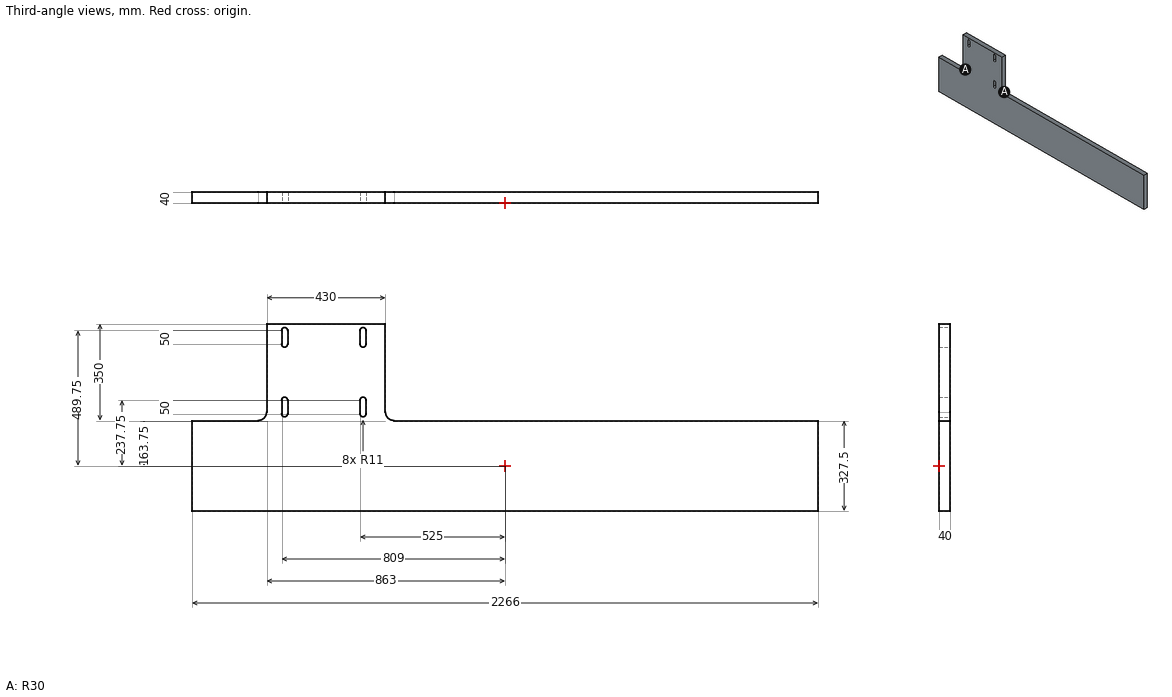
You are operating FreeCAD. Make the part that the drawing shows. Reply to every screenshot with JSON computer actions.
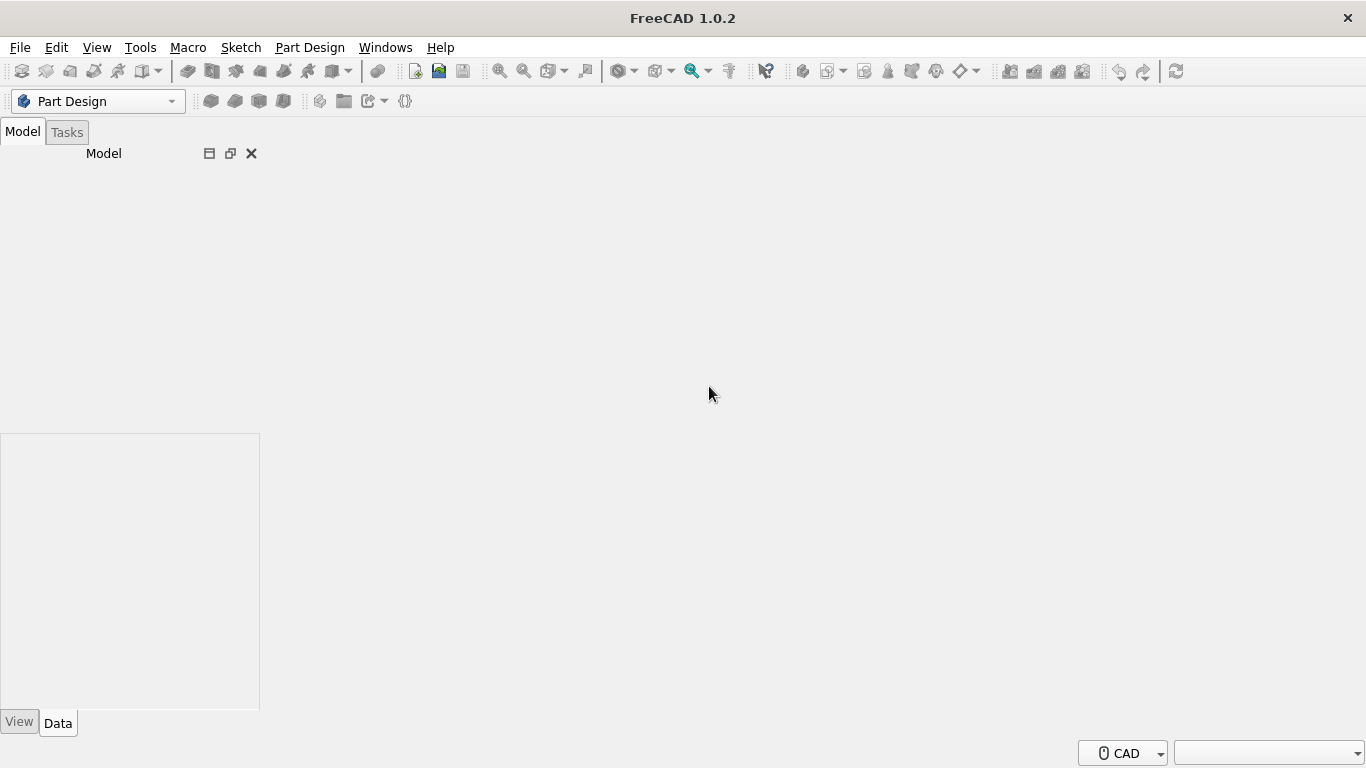
{"action": "left_click", "coordinate": [416, 72]}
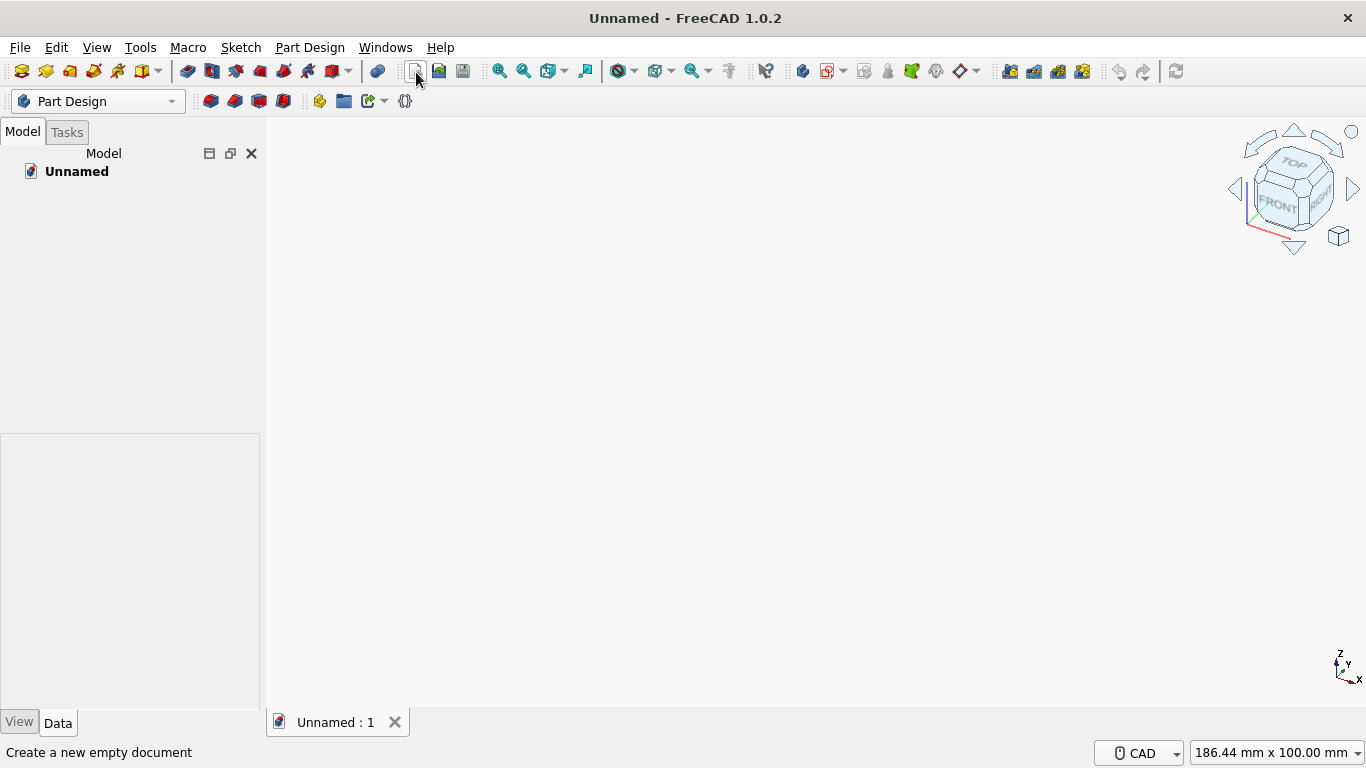
{"action": "left_click", "coordinate": [828, 72]}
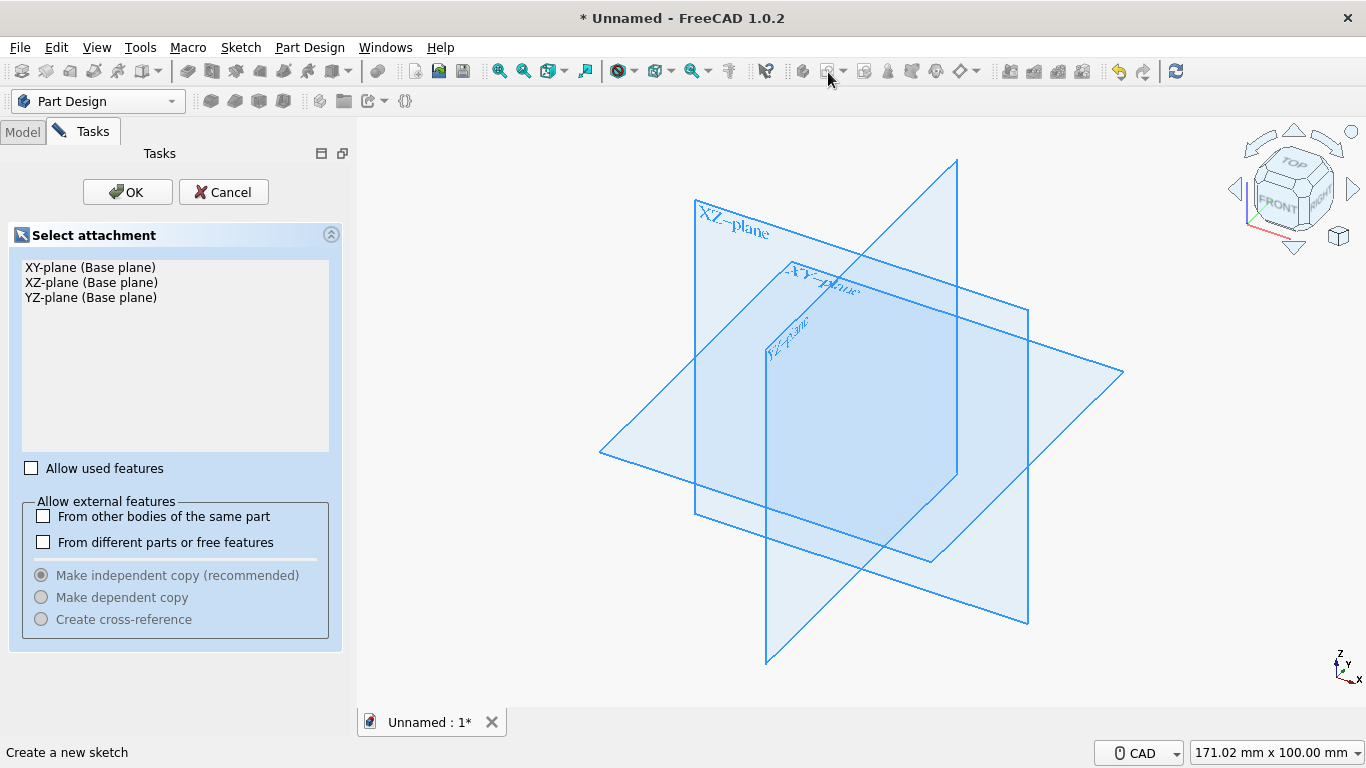
{"action": "left_click", "coordinate": [82, 282]}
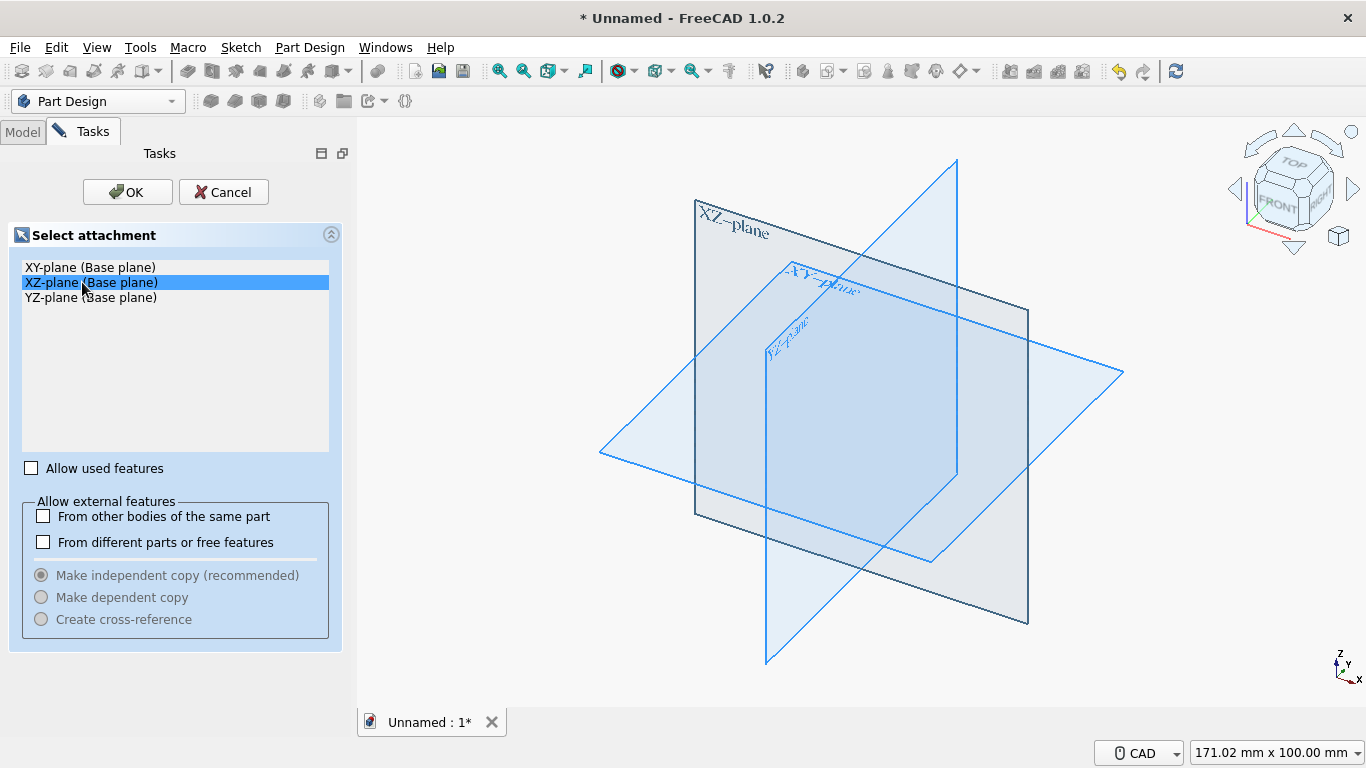
{"action": "left_click", "coordinate": [128, 192]}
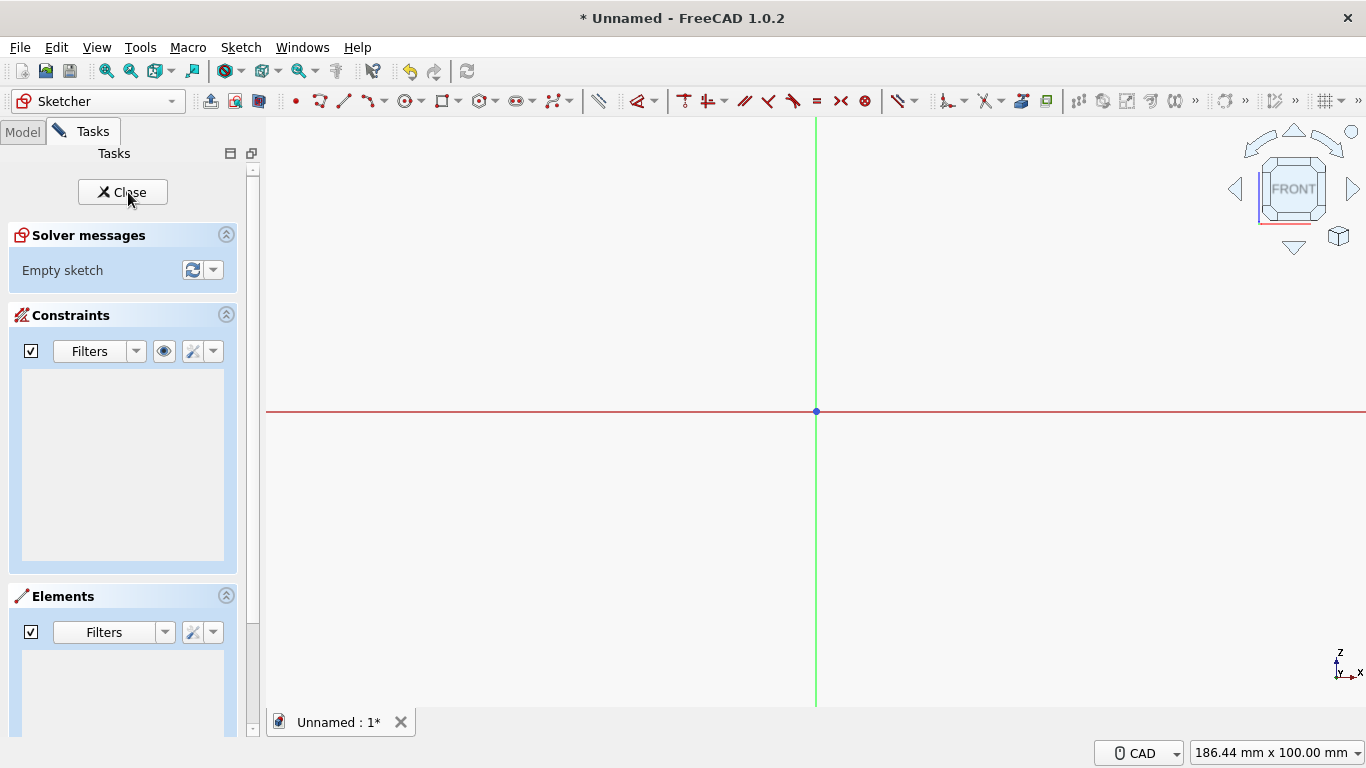
{"action": "scroll", "coordinate": [744, 412], "scroll_direction": "down", "scroll_amount": 15}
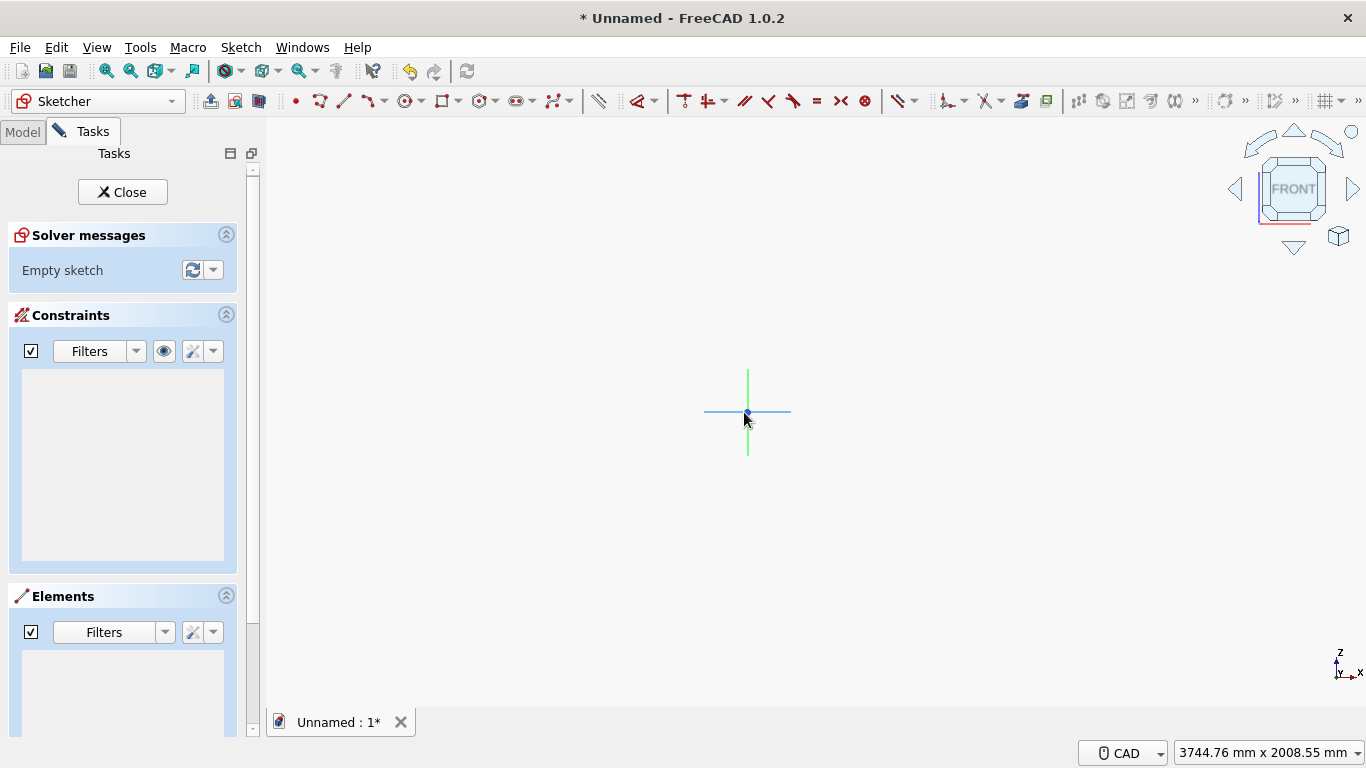
{"action": "left_click", "coordinate": [460, 102]}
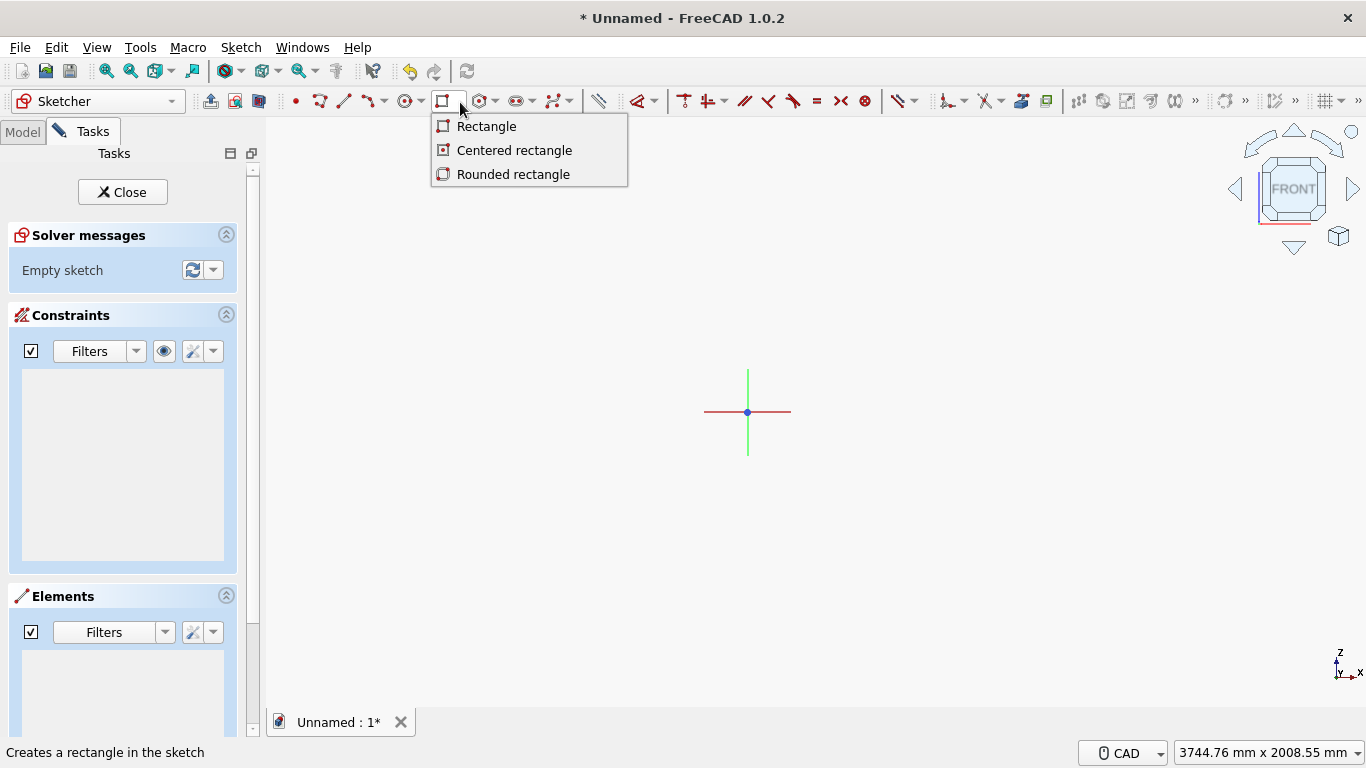
{"action": "left_click", "coordinate": [530, 150]}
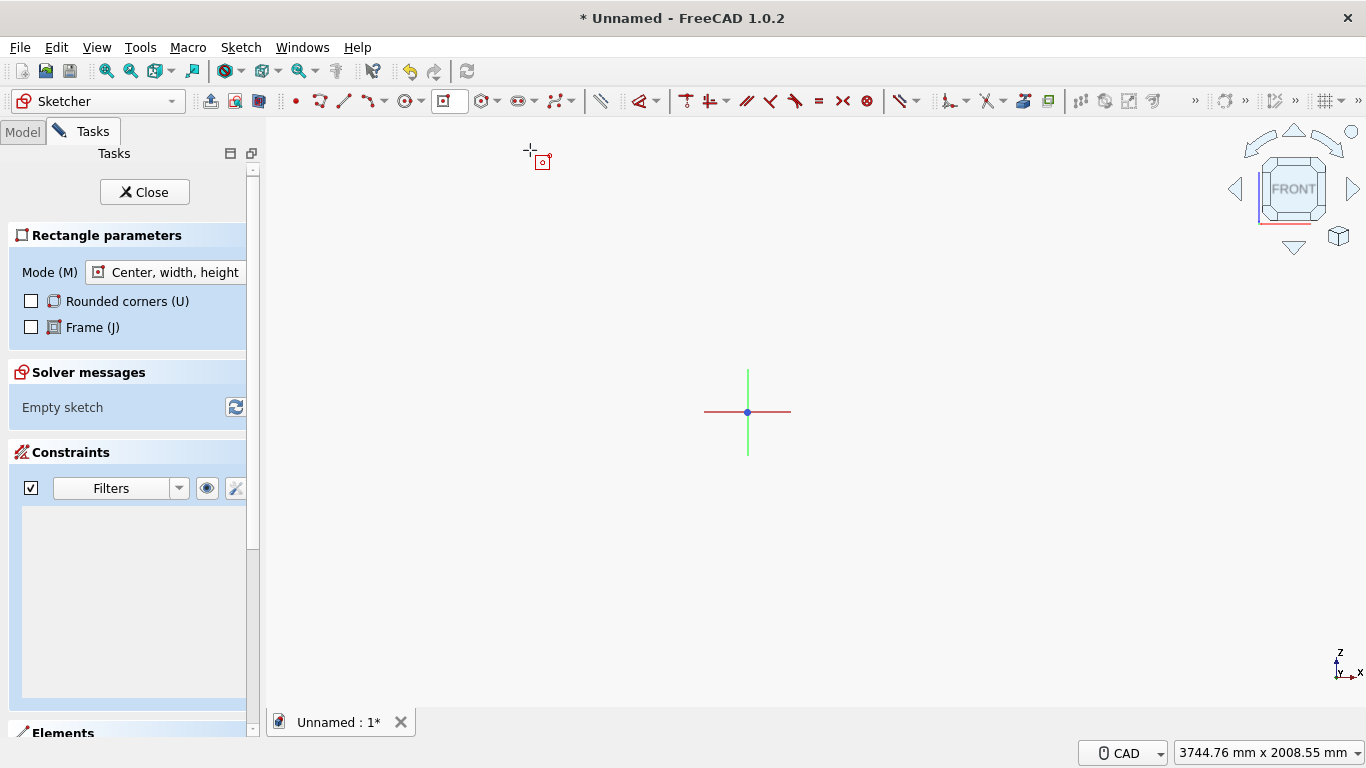
{"action": "left_click", "coordinate": [748, 412]}
{"action": "mouse_move", "coordinate": [1081, 364]}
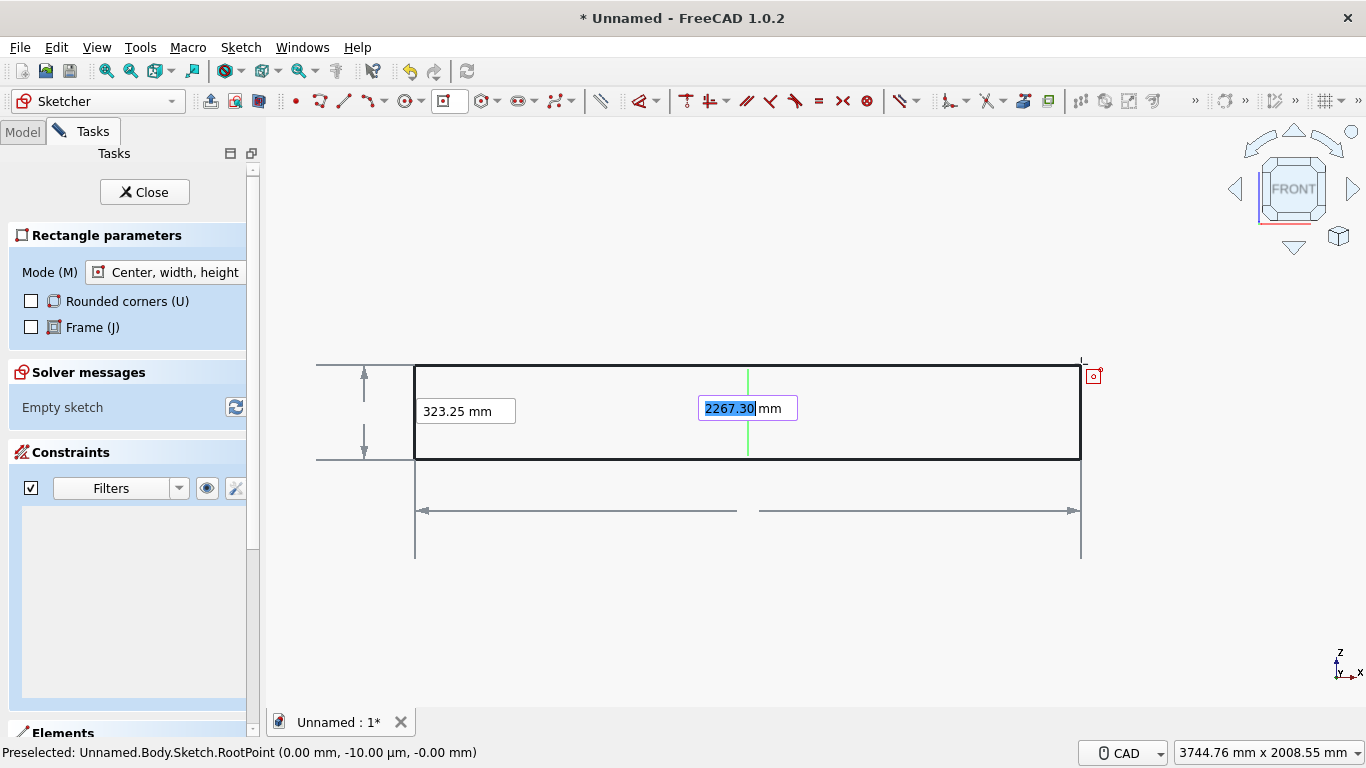
{"action": "type", "text": "2266"}
{"action": "key", "text": "Tab"}
{"action": "type", "text": "327.5"}
{"action": "key", "text": "Return"}
{"action": "key", "text": "Escape"}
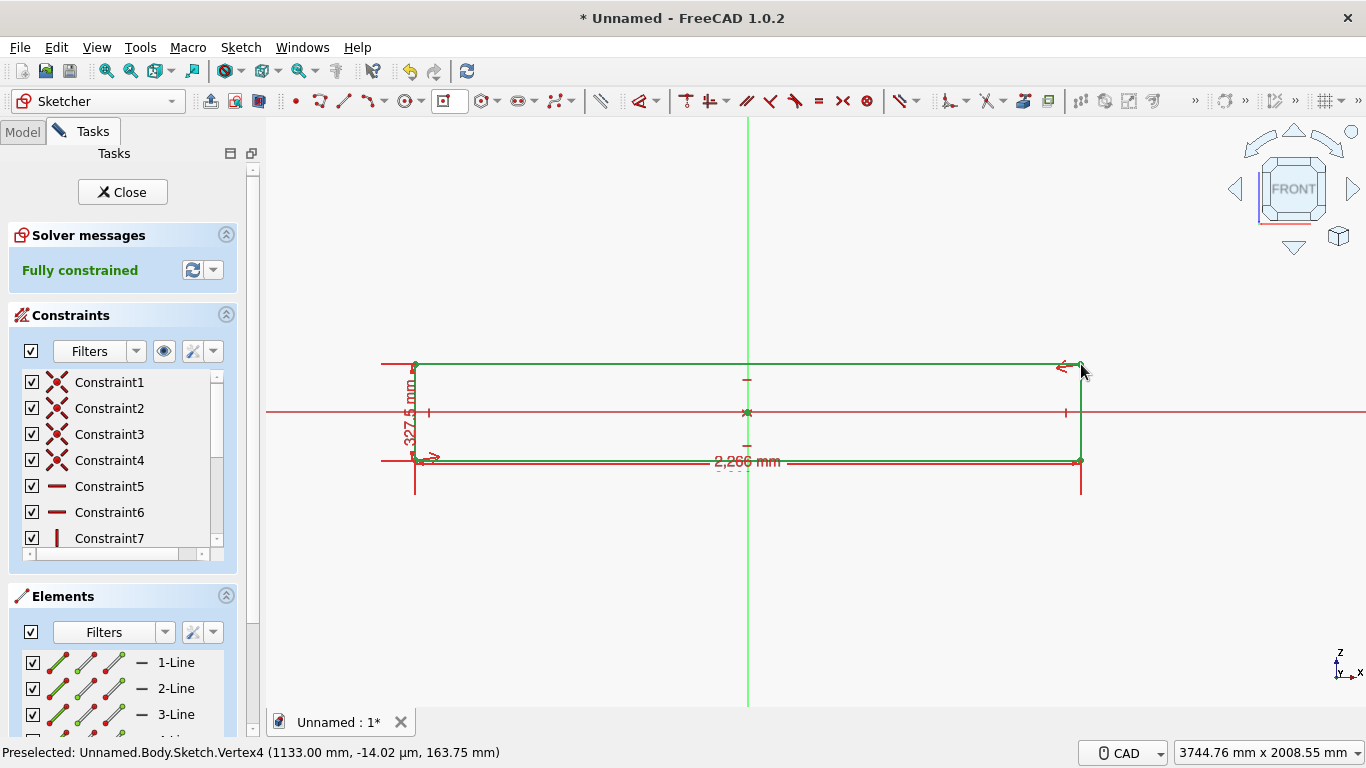
{"action": "left_click", "coordinate": [123, 192]}